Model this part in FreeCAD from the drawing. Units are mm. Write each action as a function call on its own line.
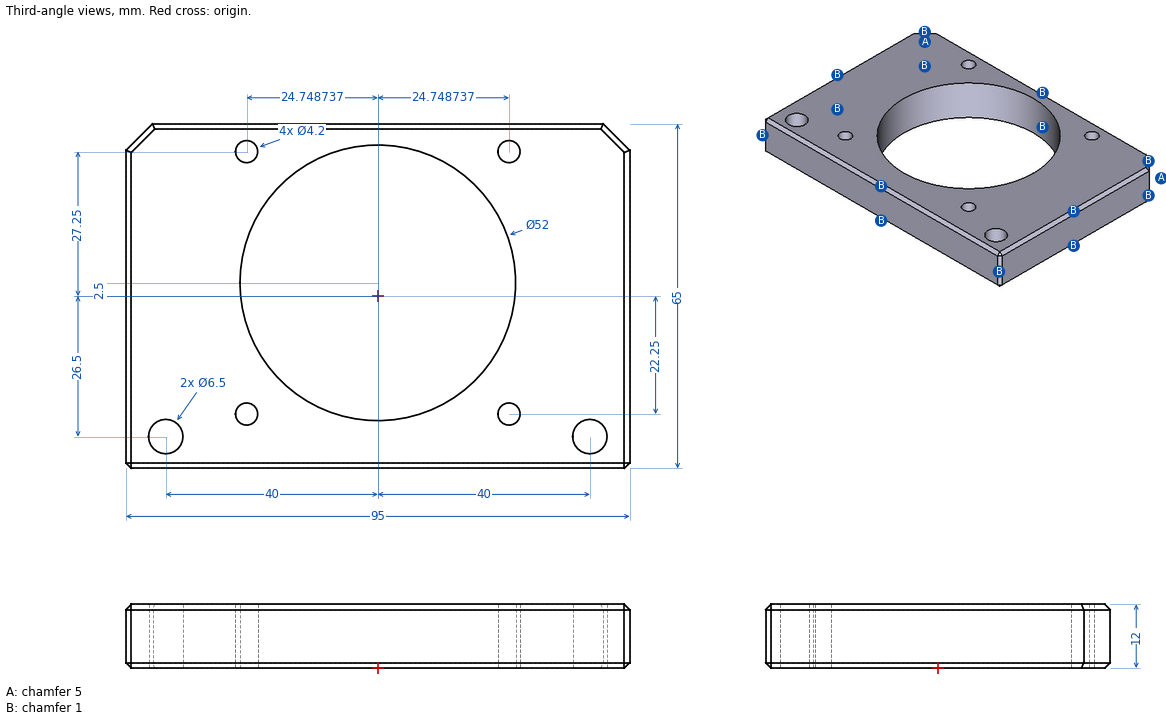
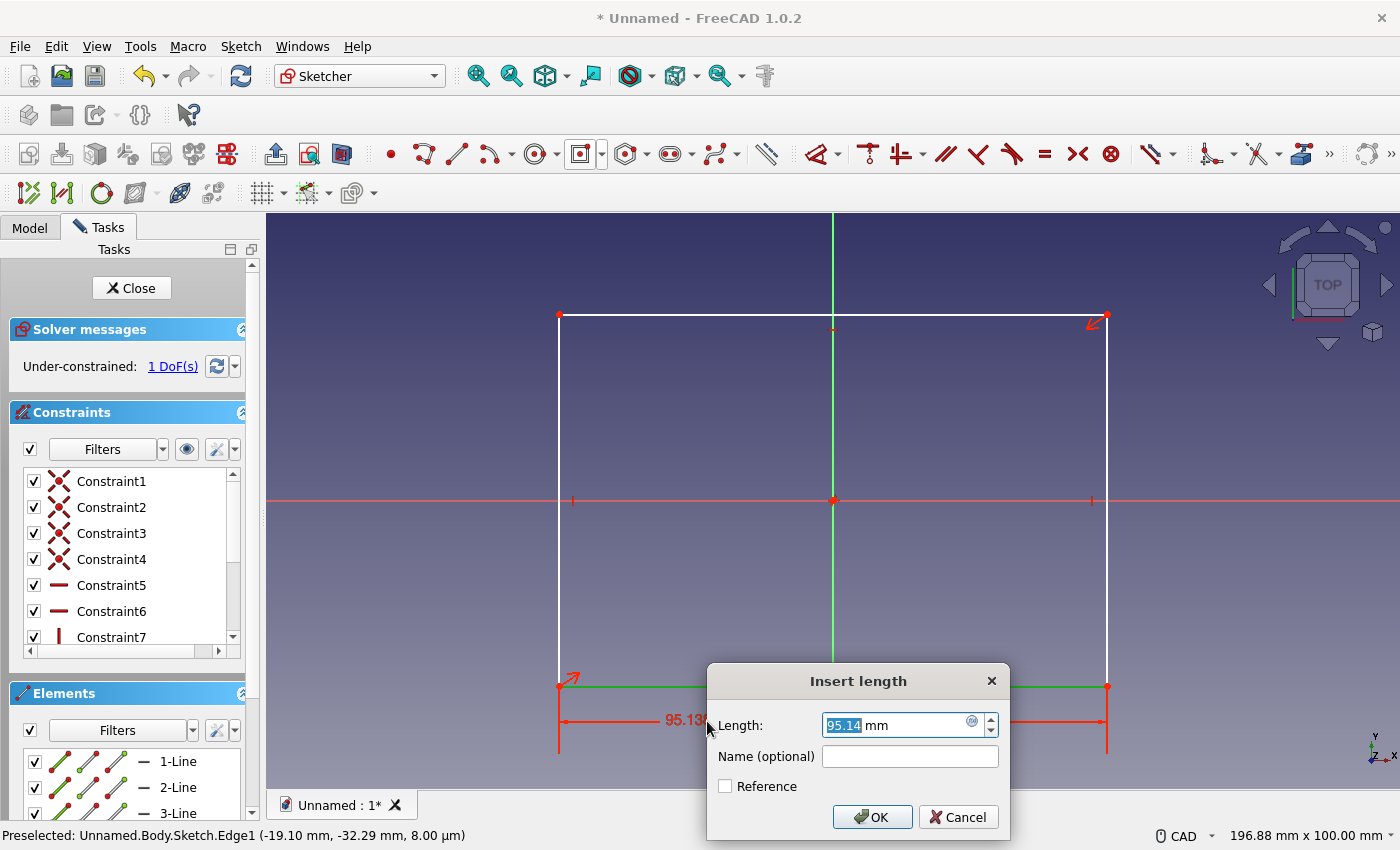
text(95)
key(Return)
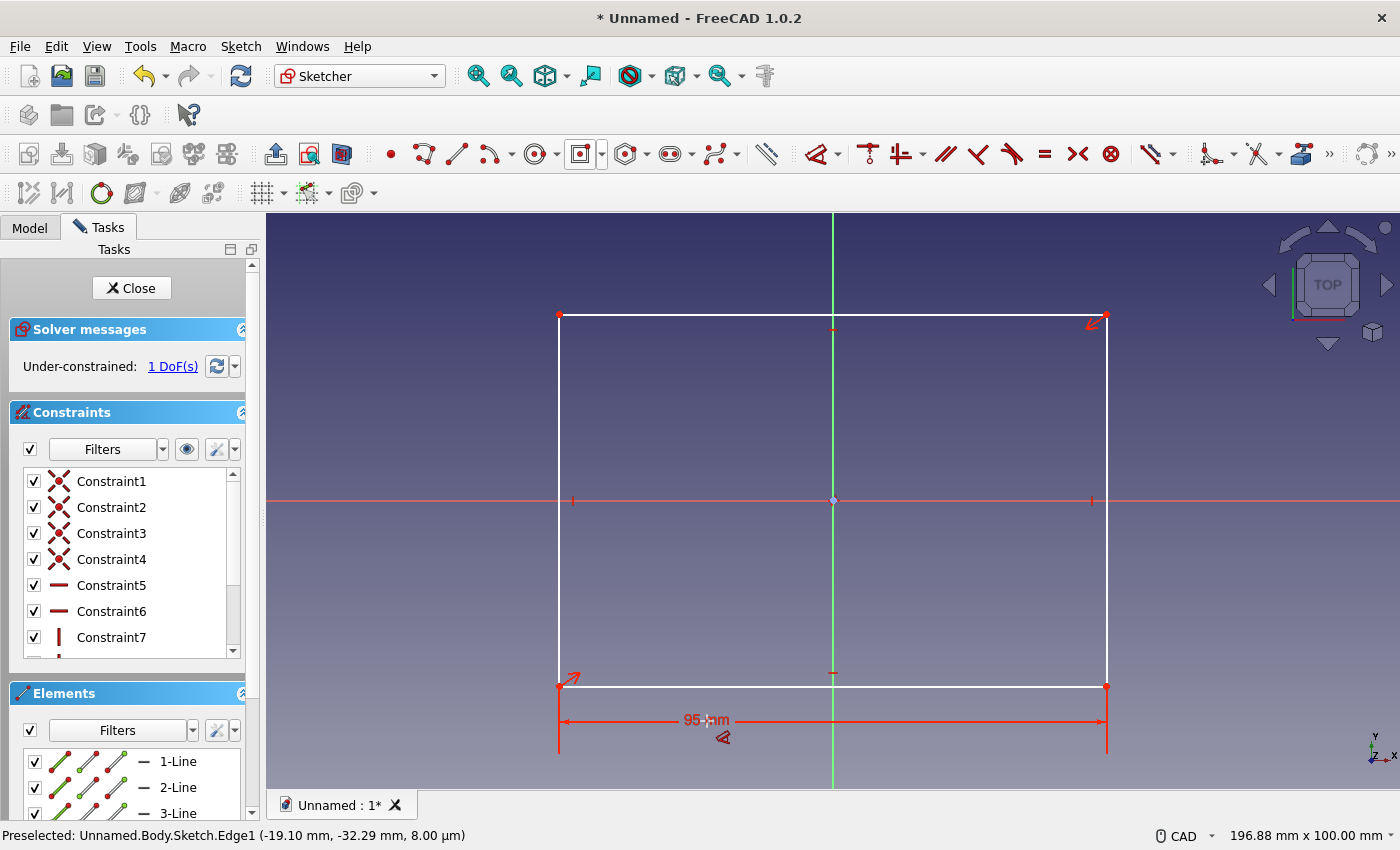
click(1107, 575)
click(1141, 415)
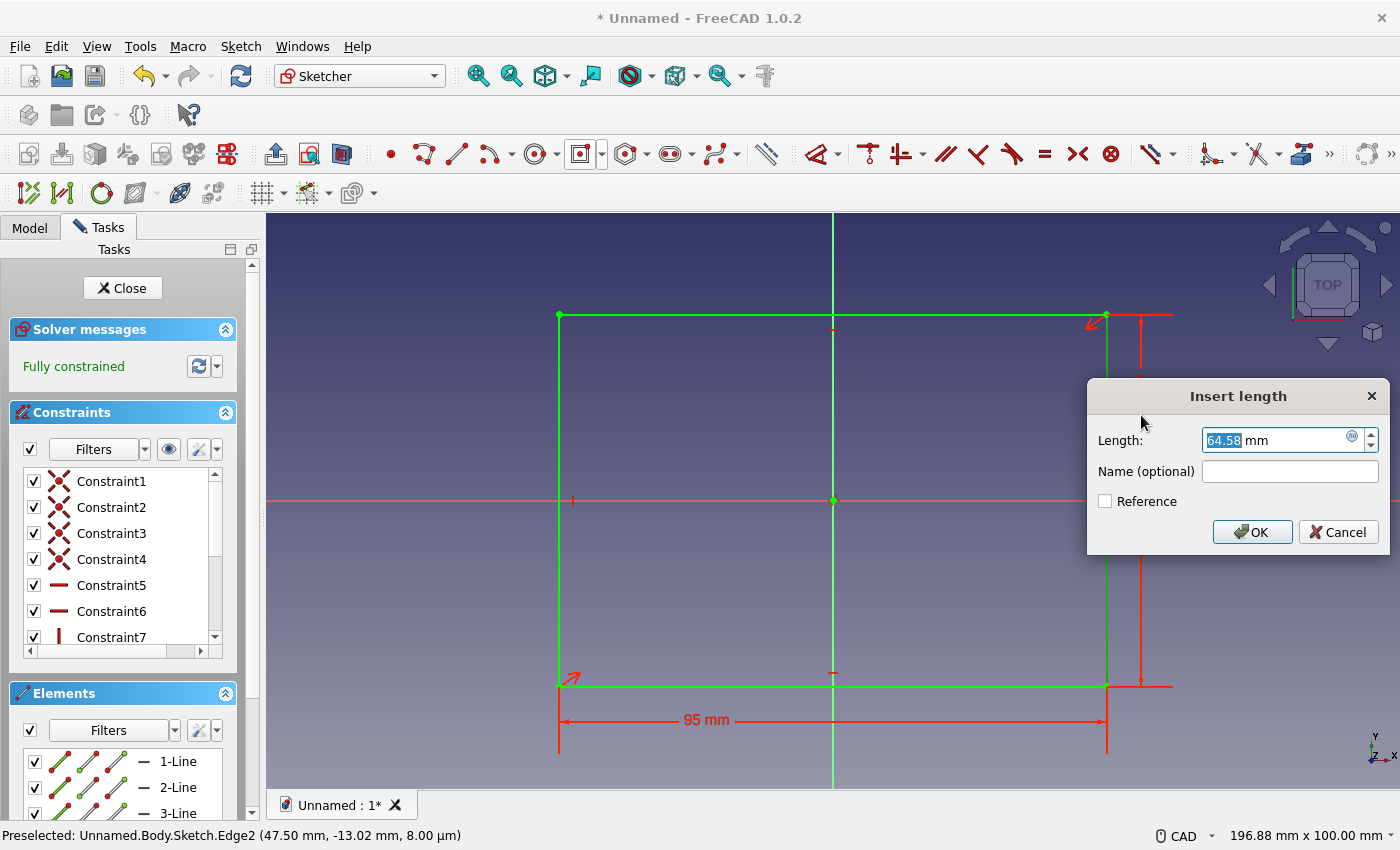
text(65)
key(Return)
key(Escape)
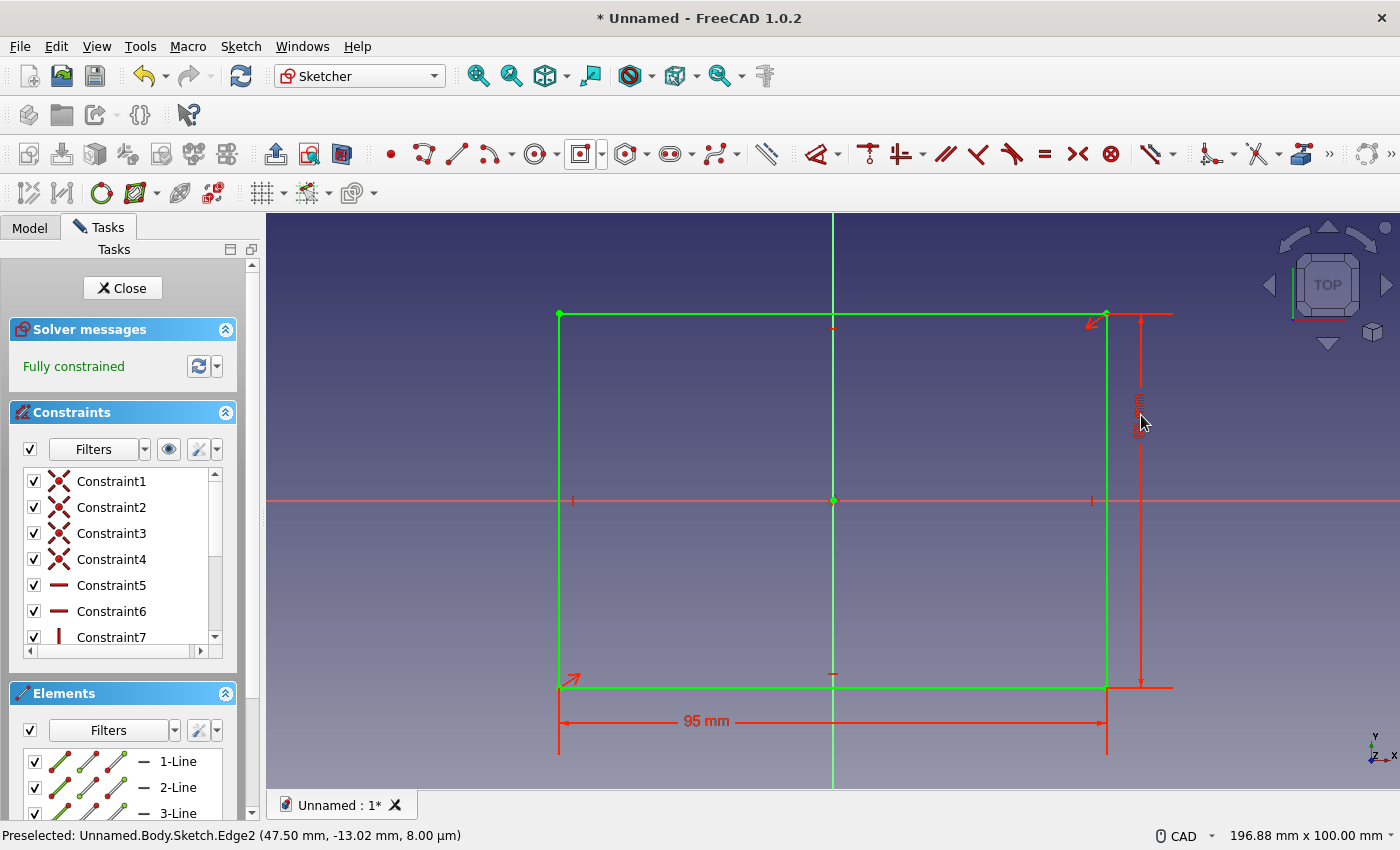
click(123, 288)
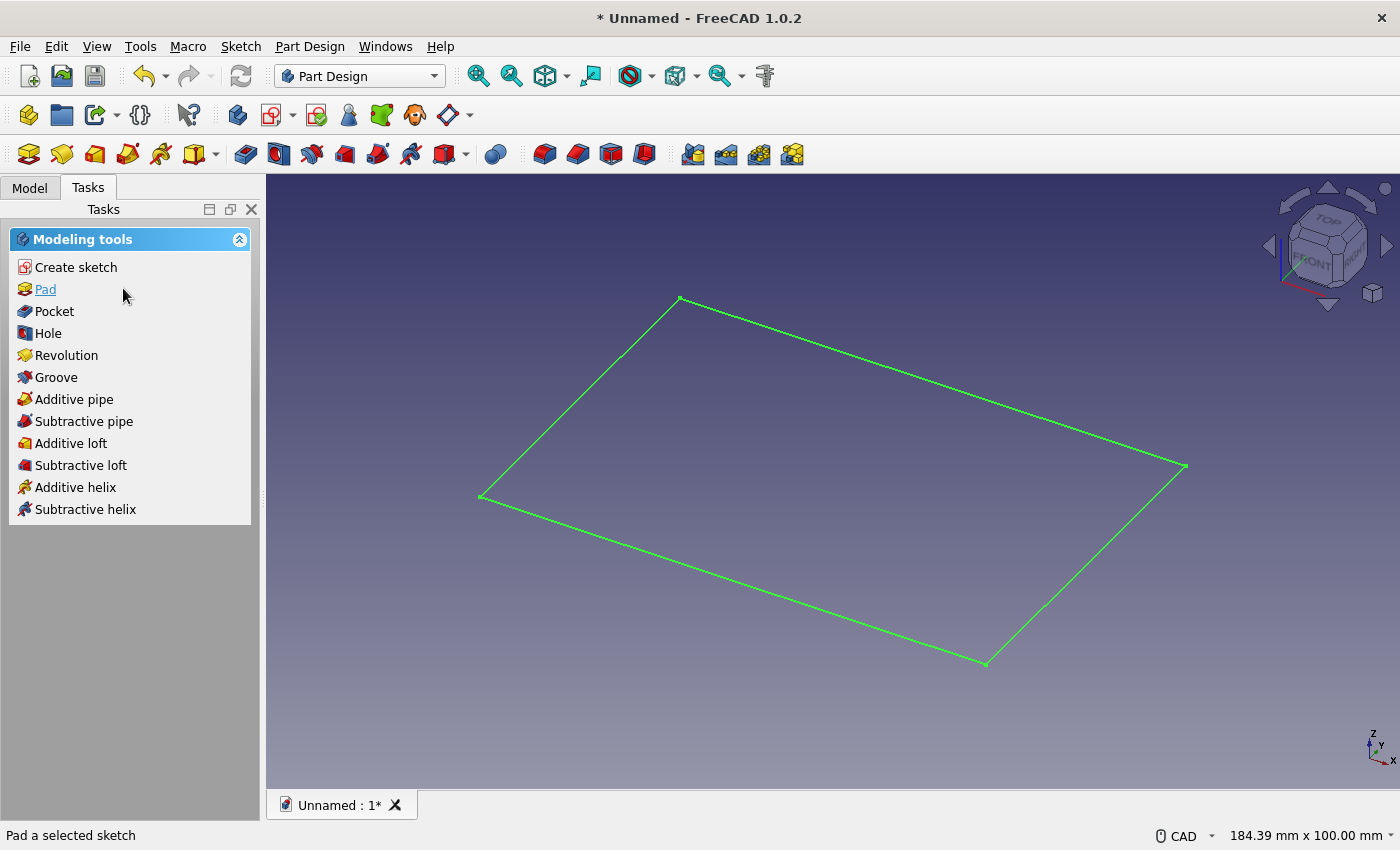
click(29, 154)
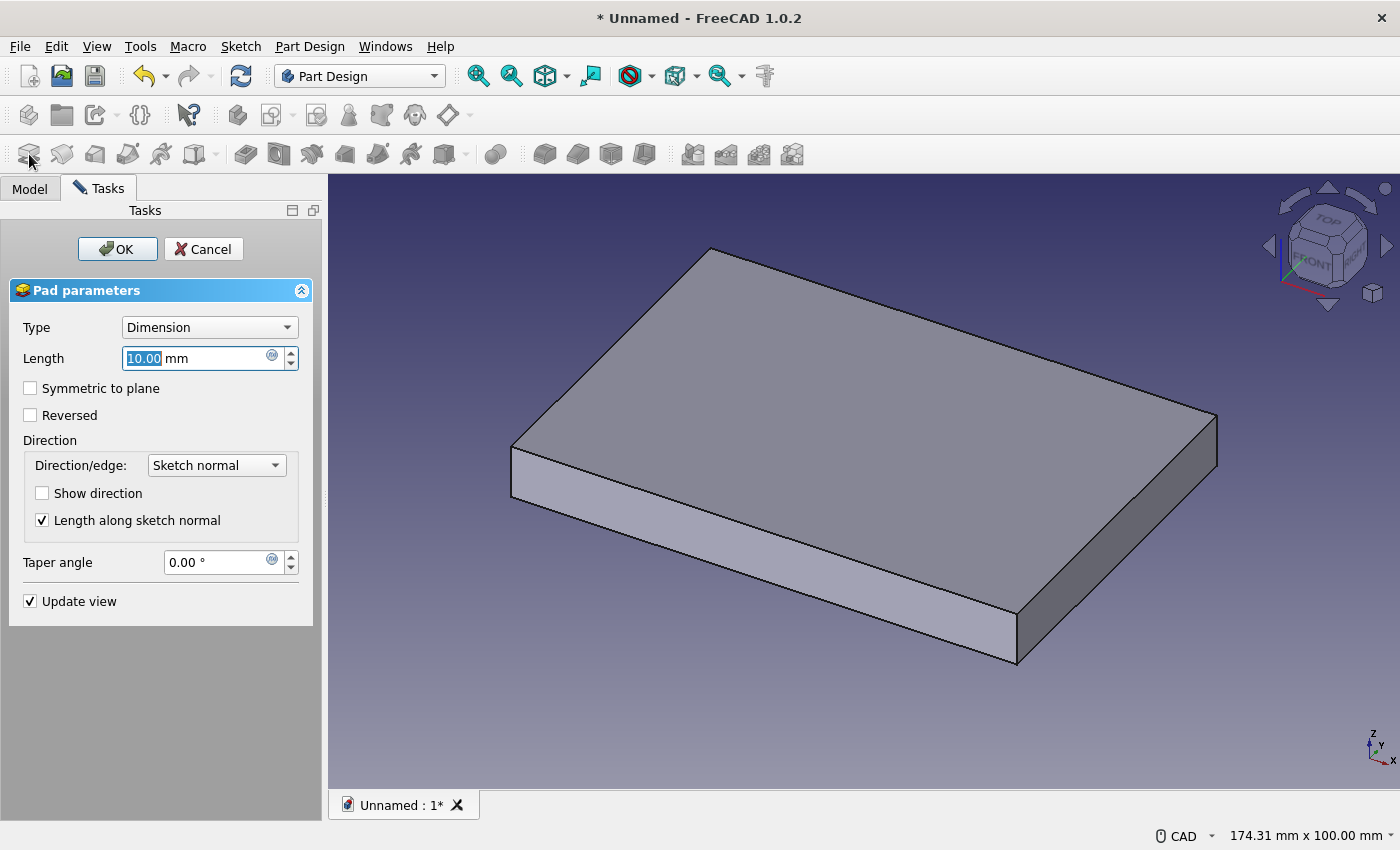
text(12)
key(Tab)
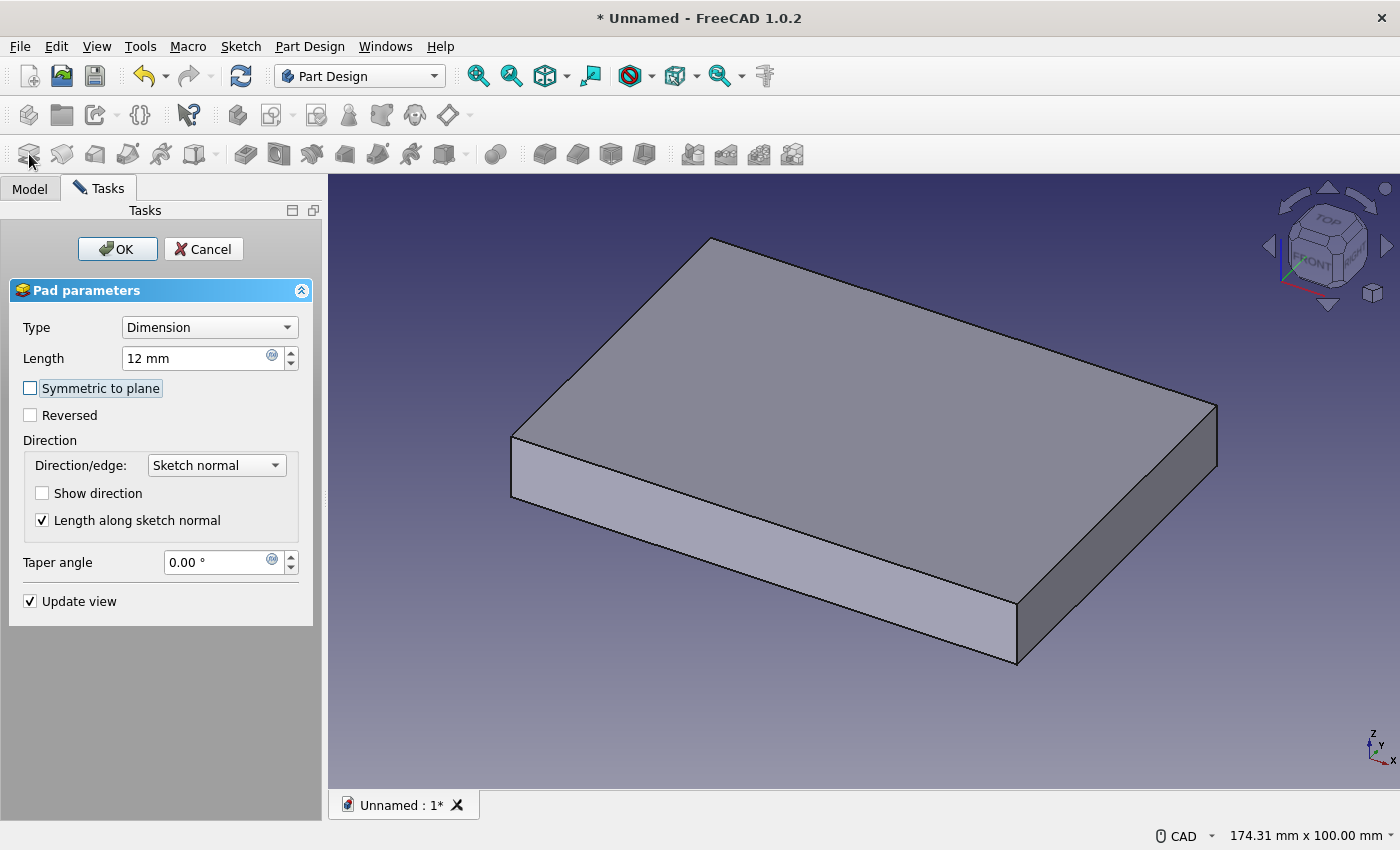
click(118, 249)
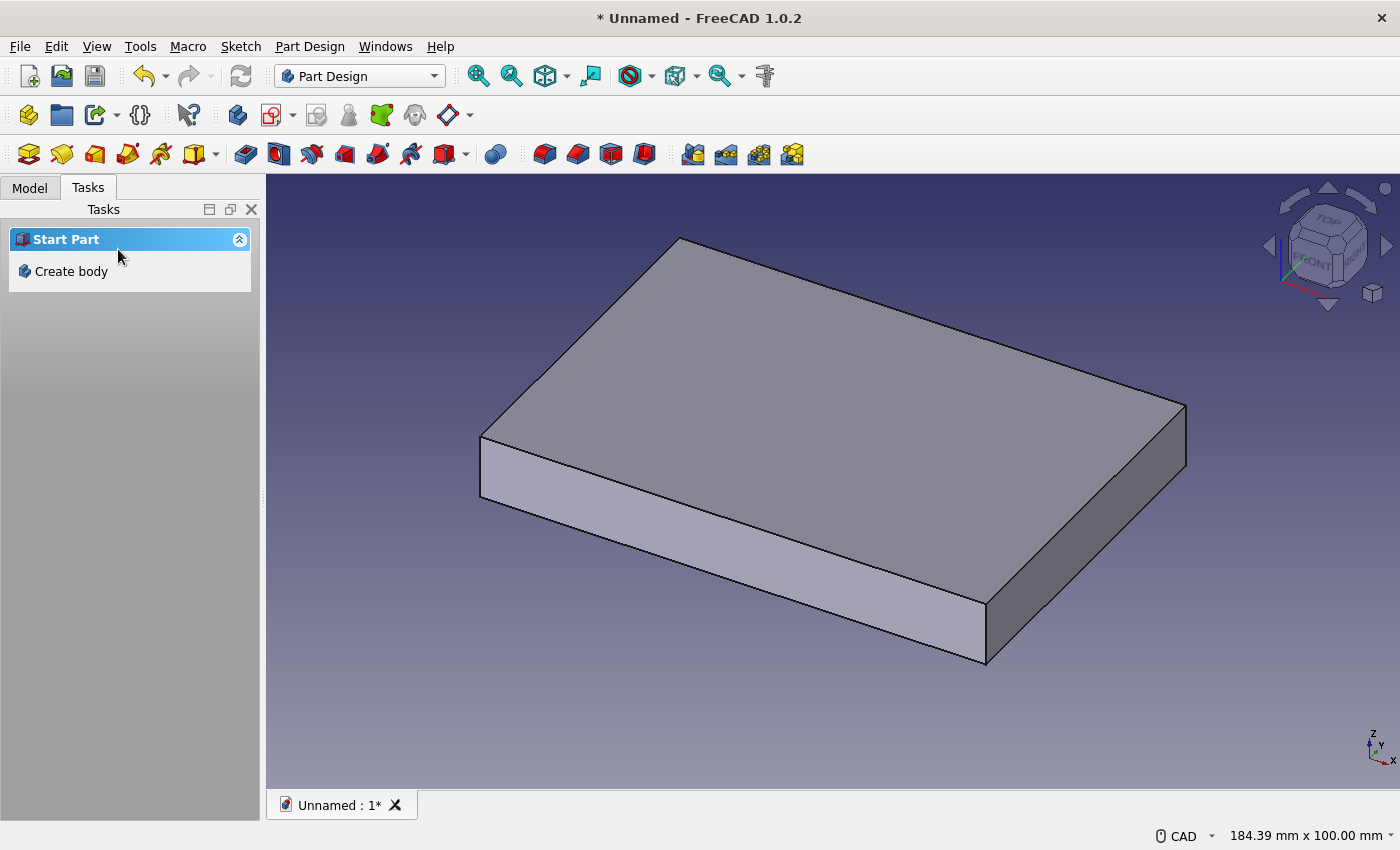
click(905, 444)